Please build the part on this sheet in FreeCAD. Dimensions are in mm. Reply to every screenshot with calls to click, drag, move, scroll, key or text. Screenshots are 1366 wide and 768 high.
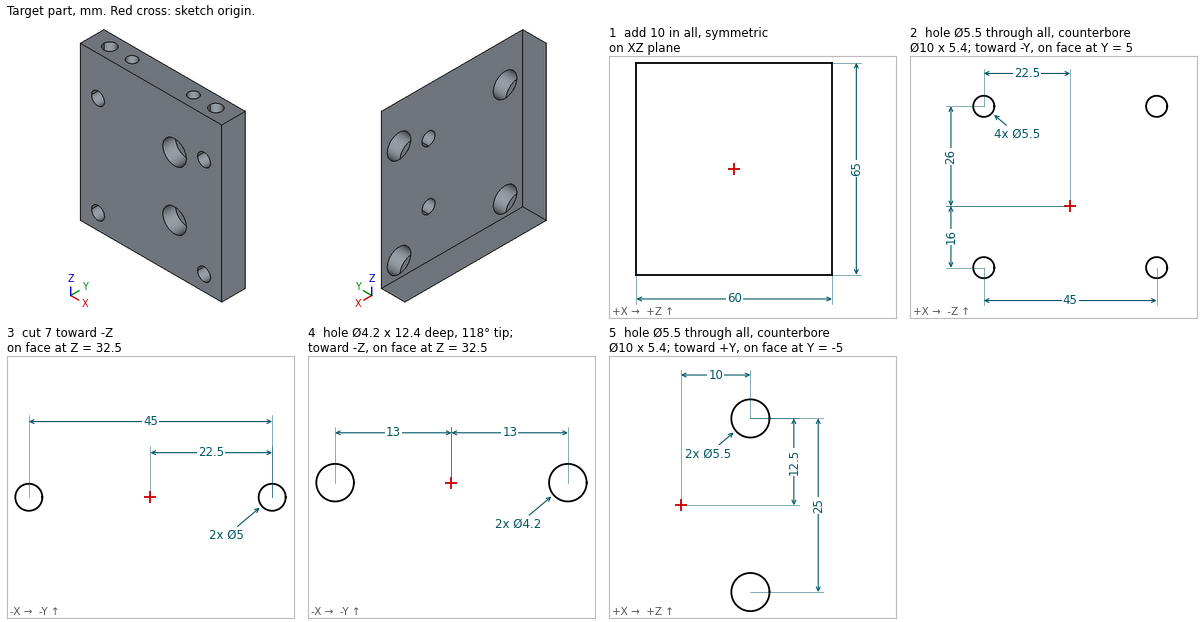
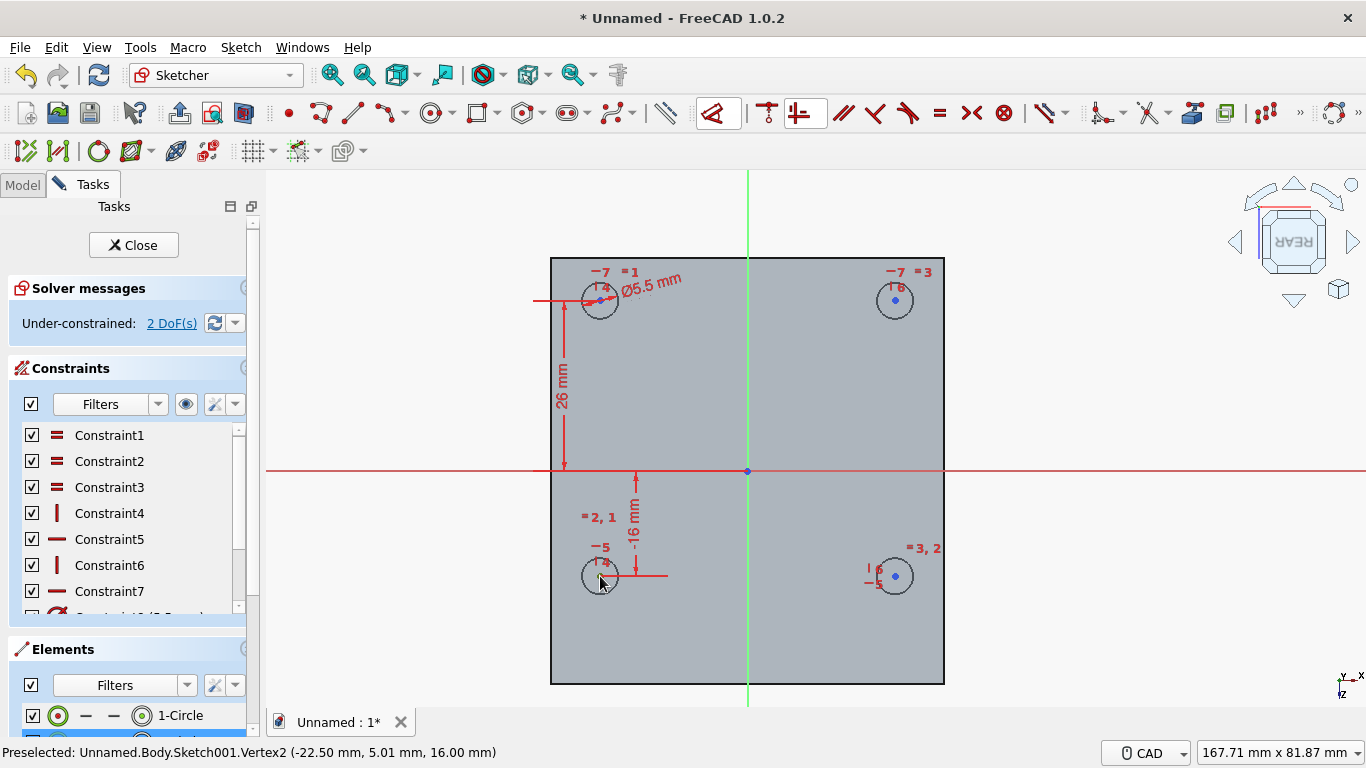
click(895, 576)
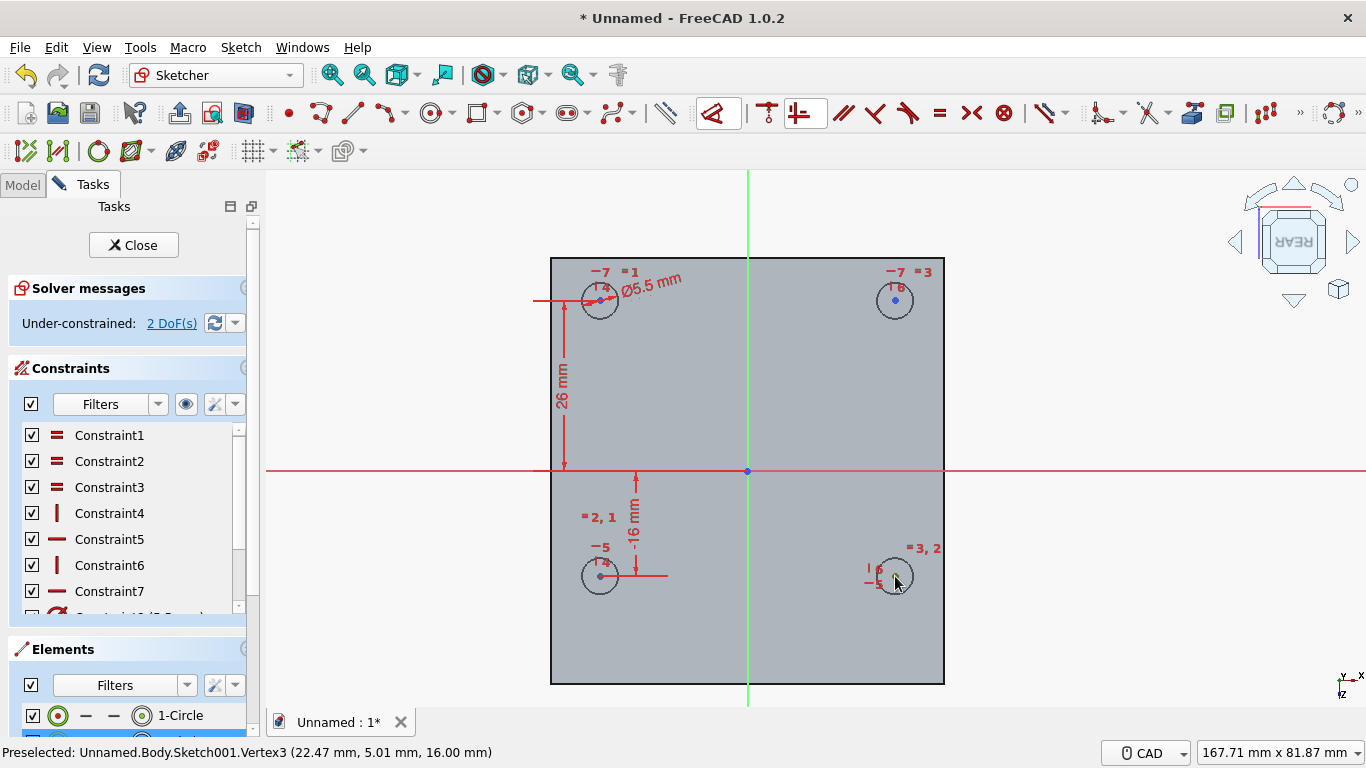
key(l)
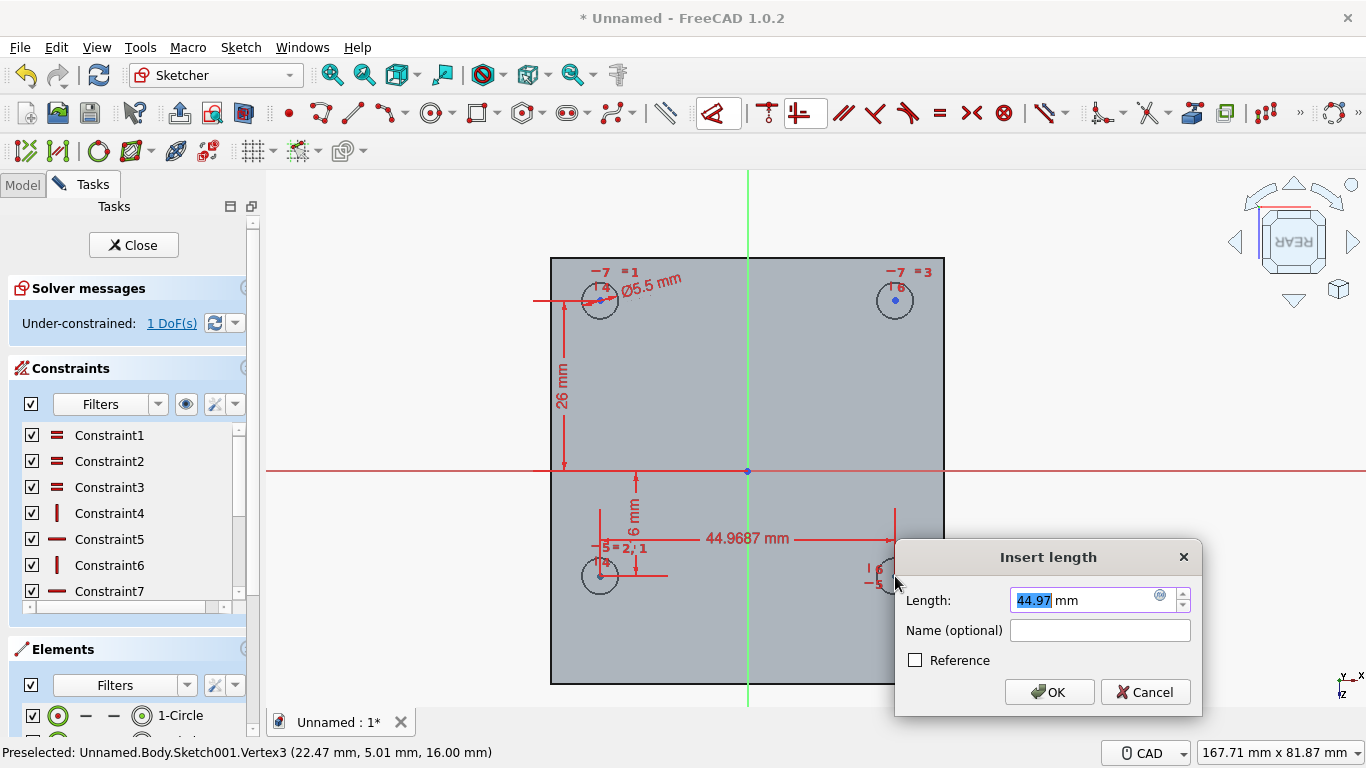
text(45)
key(Return)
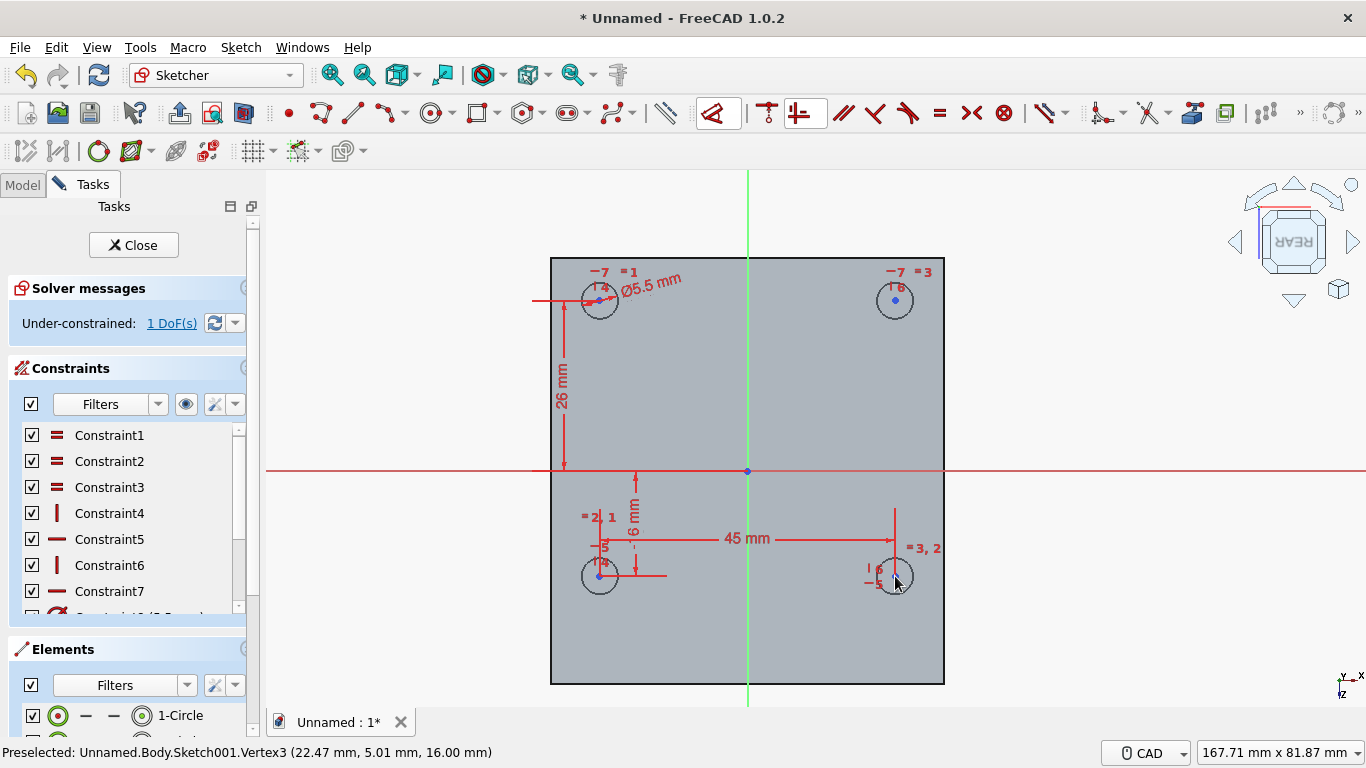
click(600, 301)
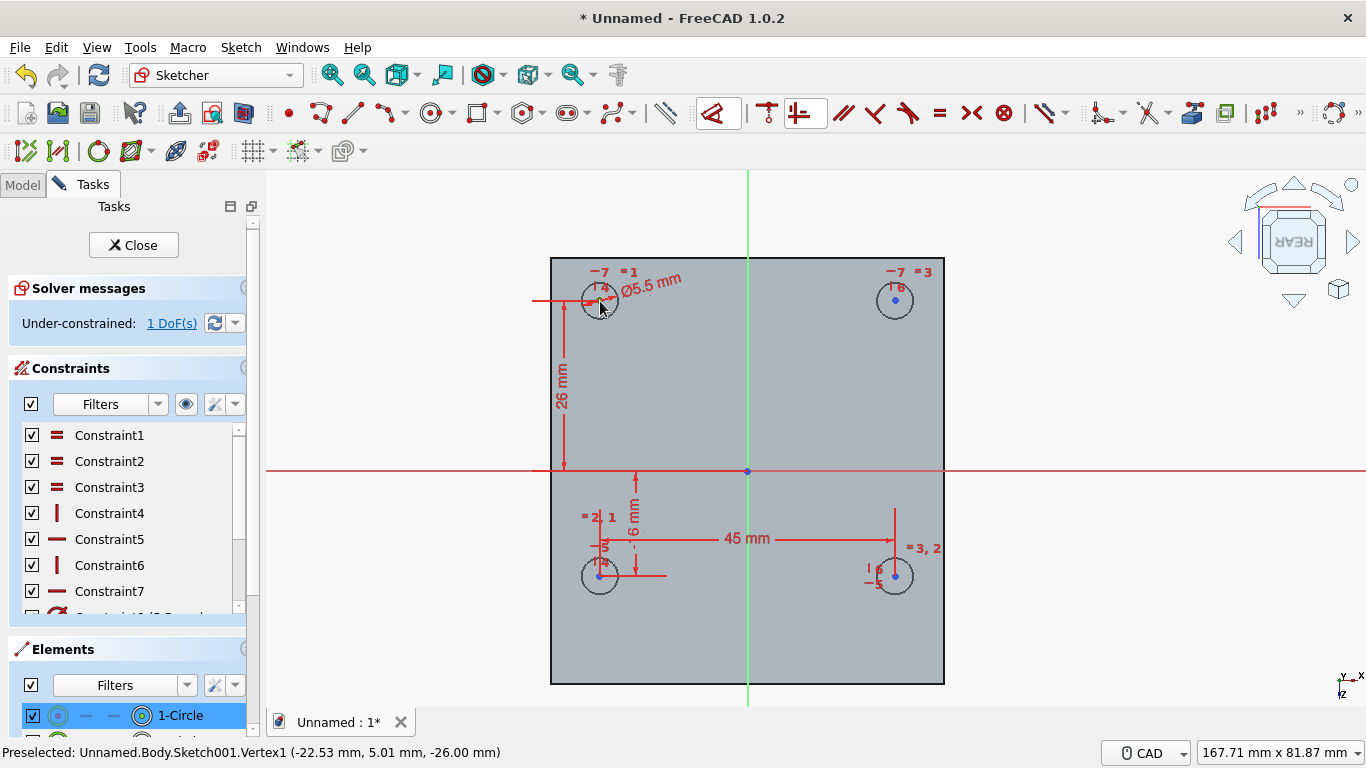
click(736, 114)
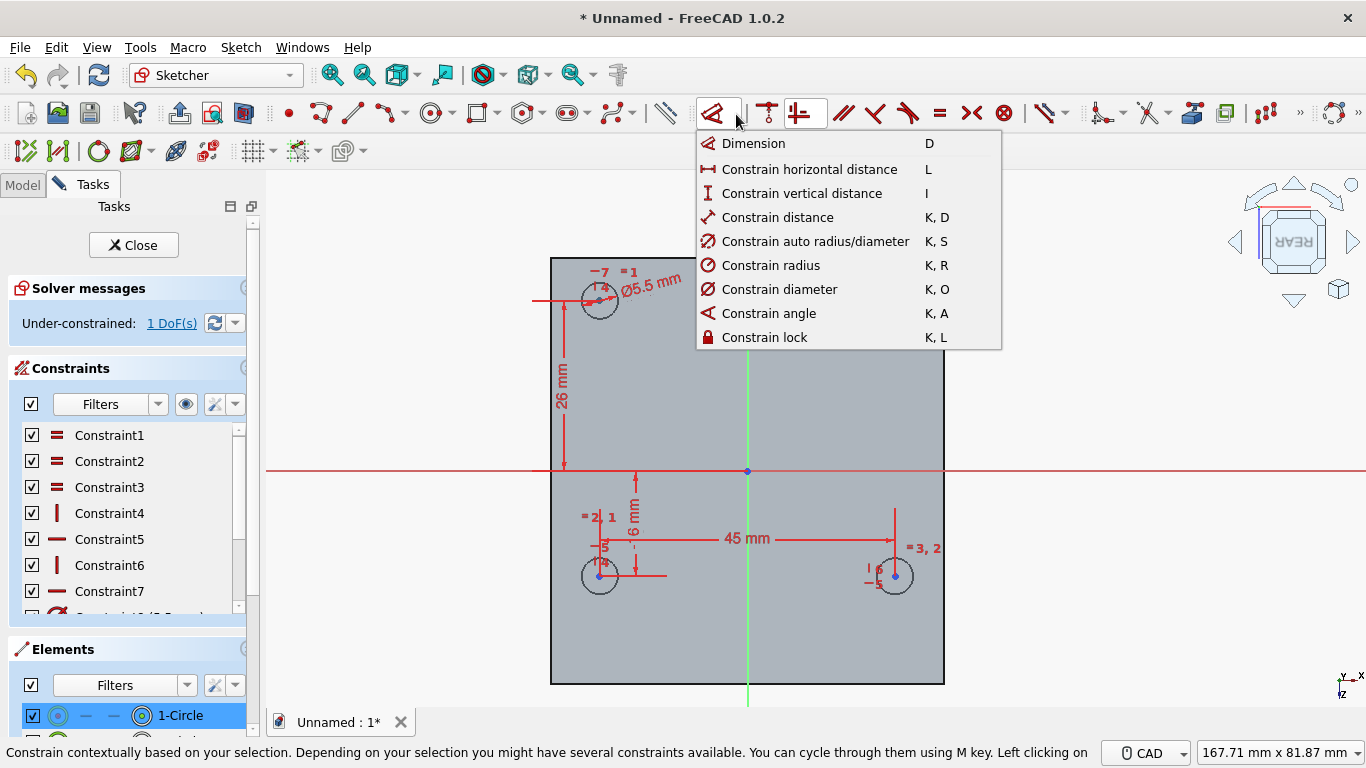
click(849, 169)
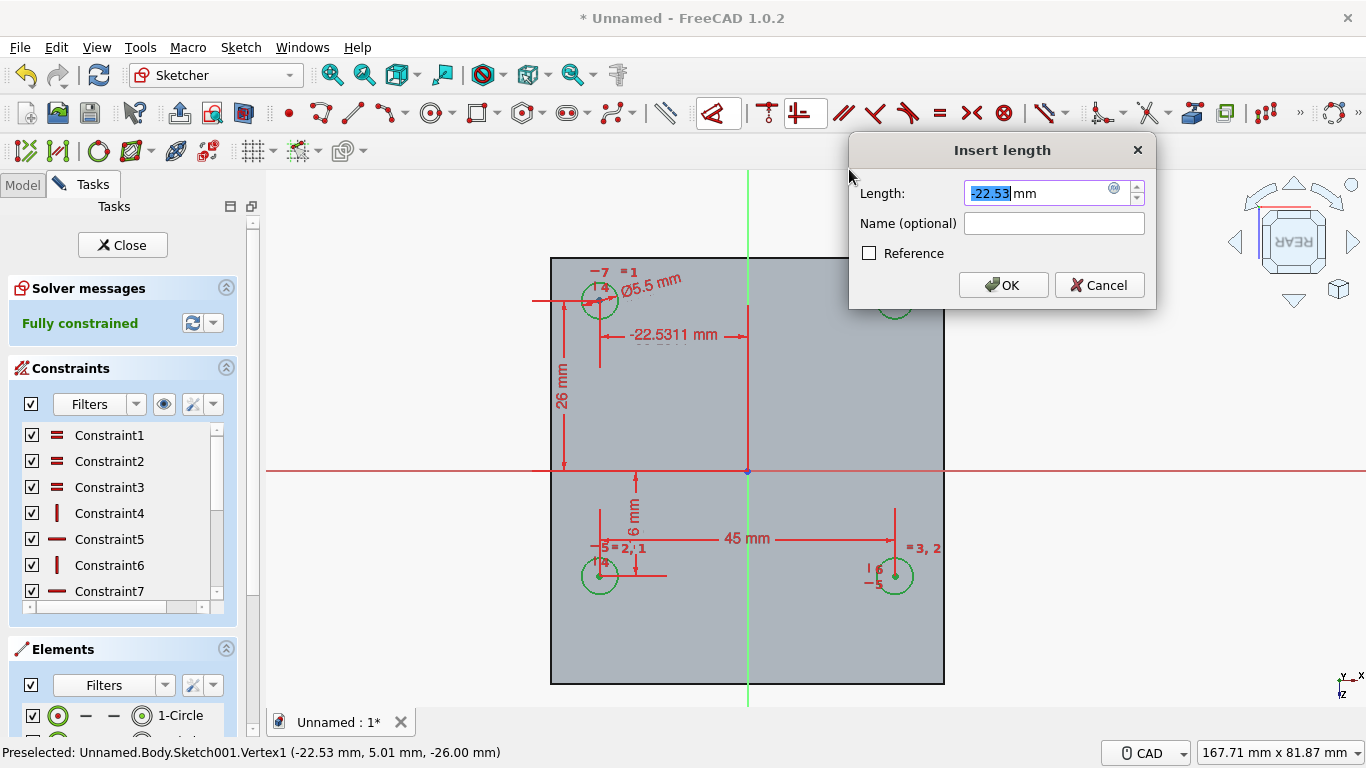
text(-22.5)
key(Return)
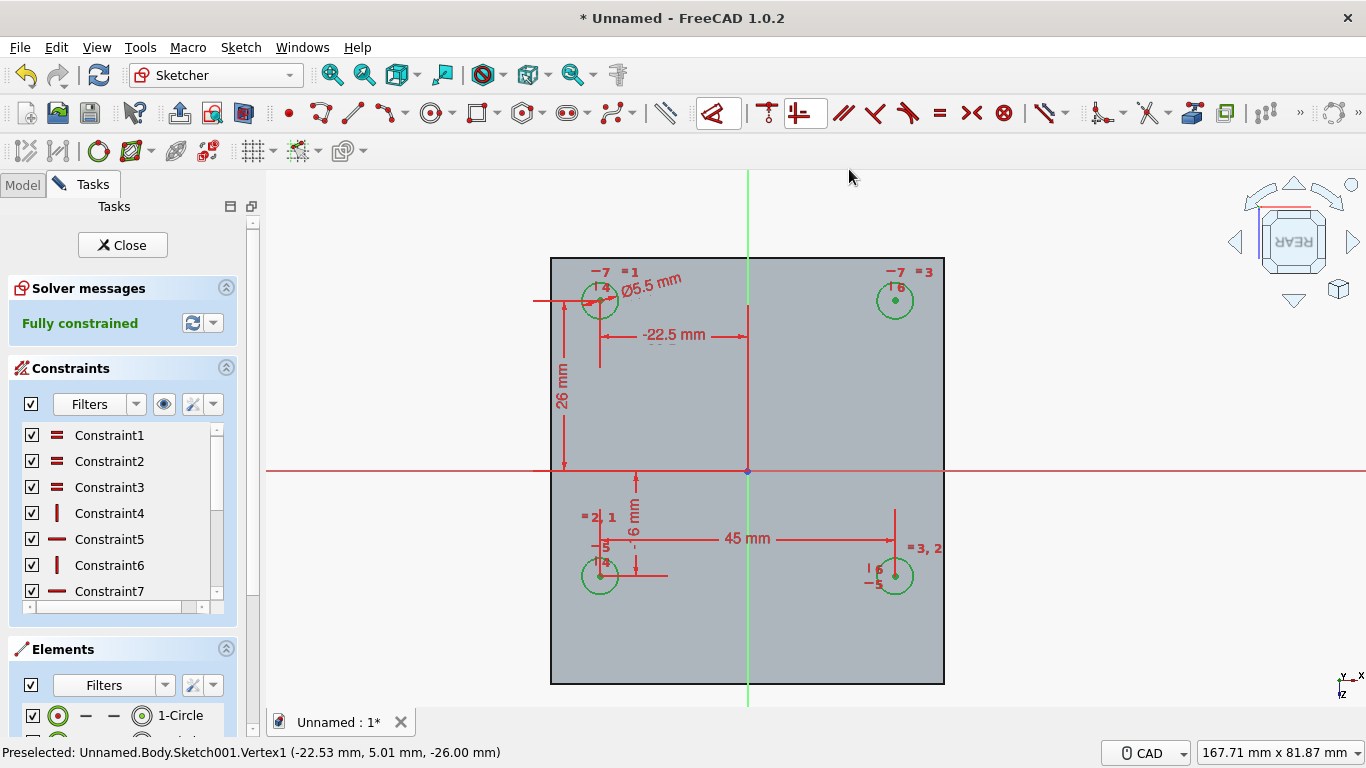
click(123, 245)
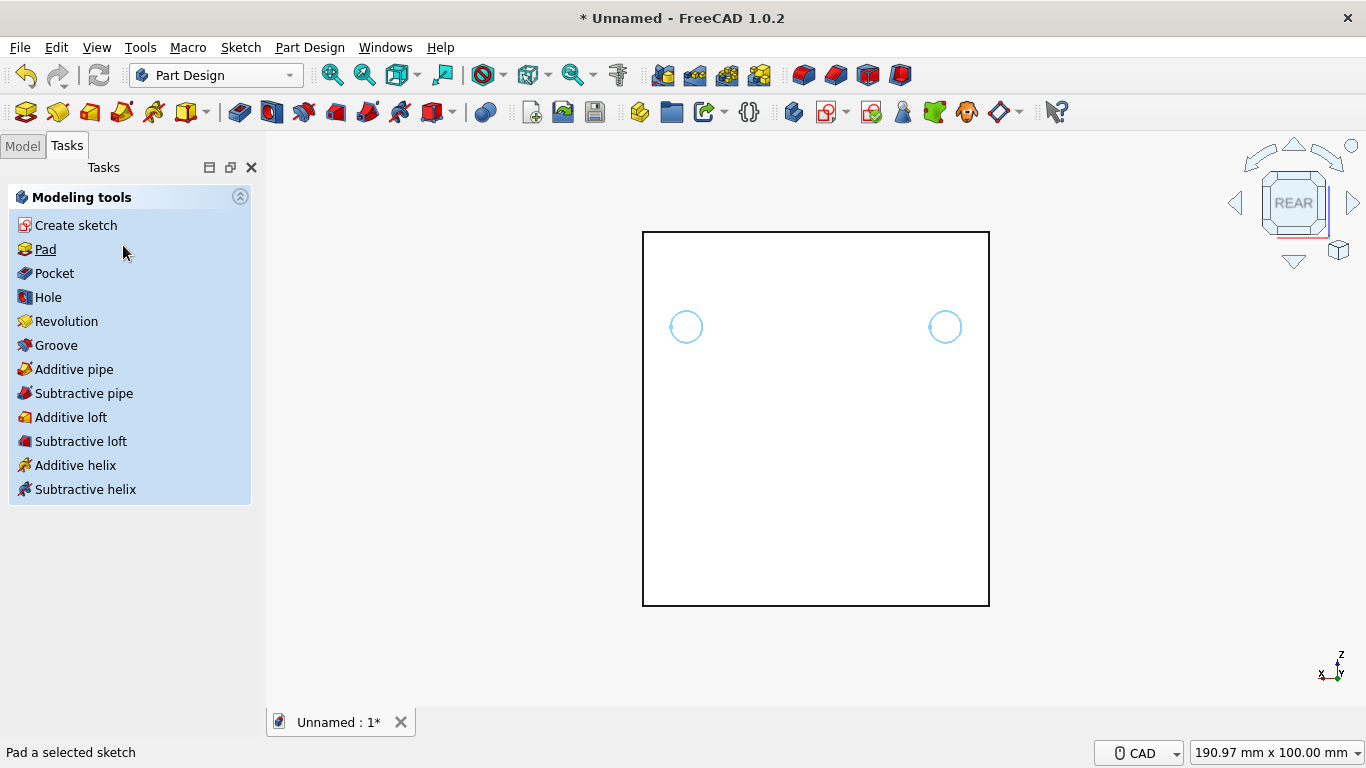
click(272, 112)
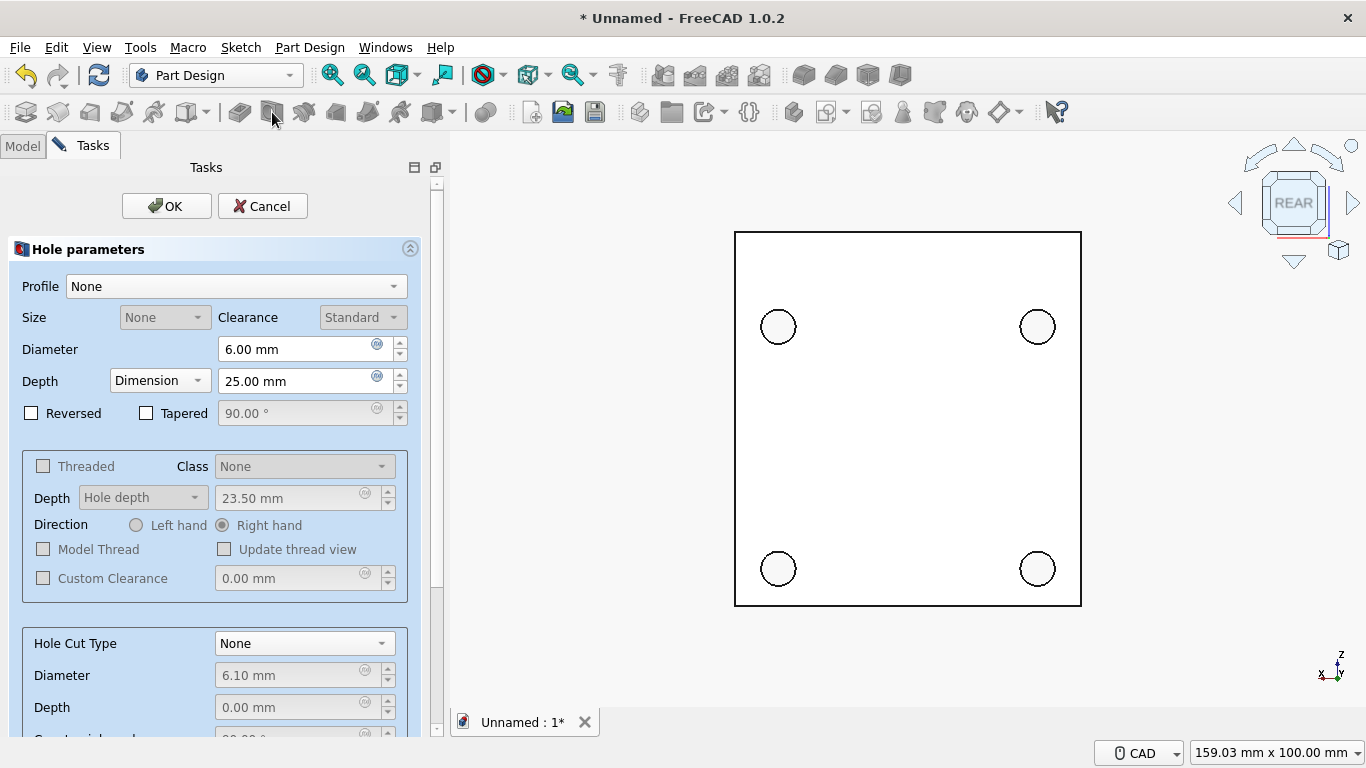
triple_click(305, 349)